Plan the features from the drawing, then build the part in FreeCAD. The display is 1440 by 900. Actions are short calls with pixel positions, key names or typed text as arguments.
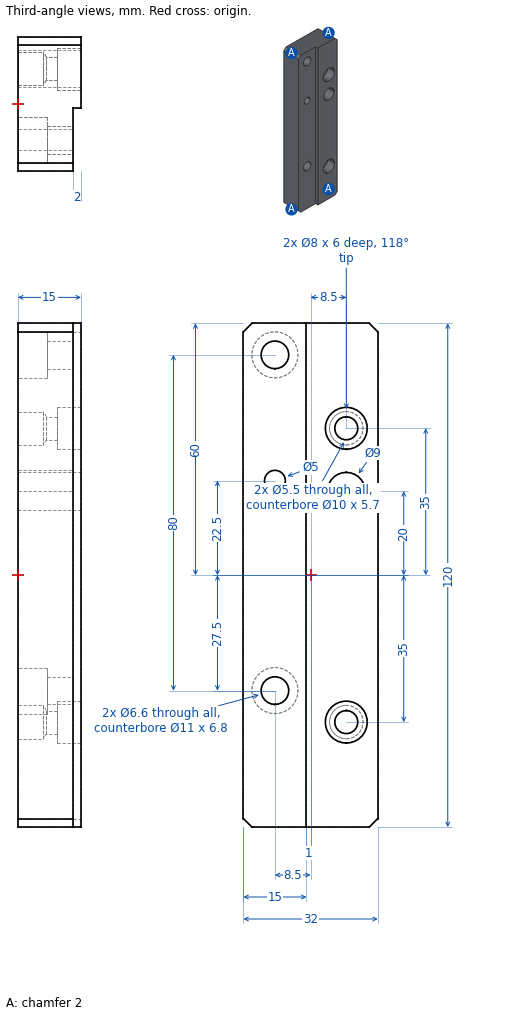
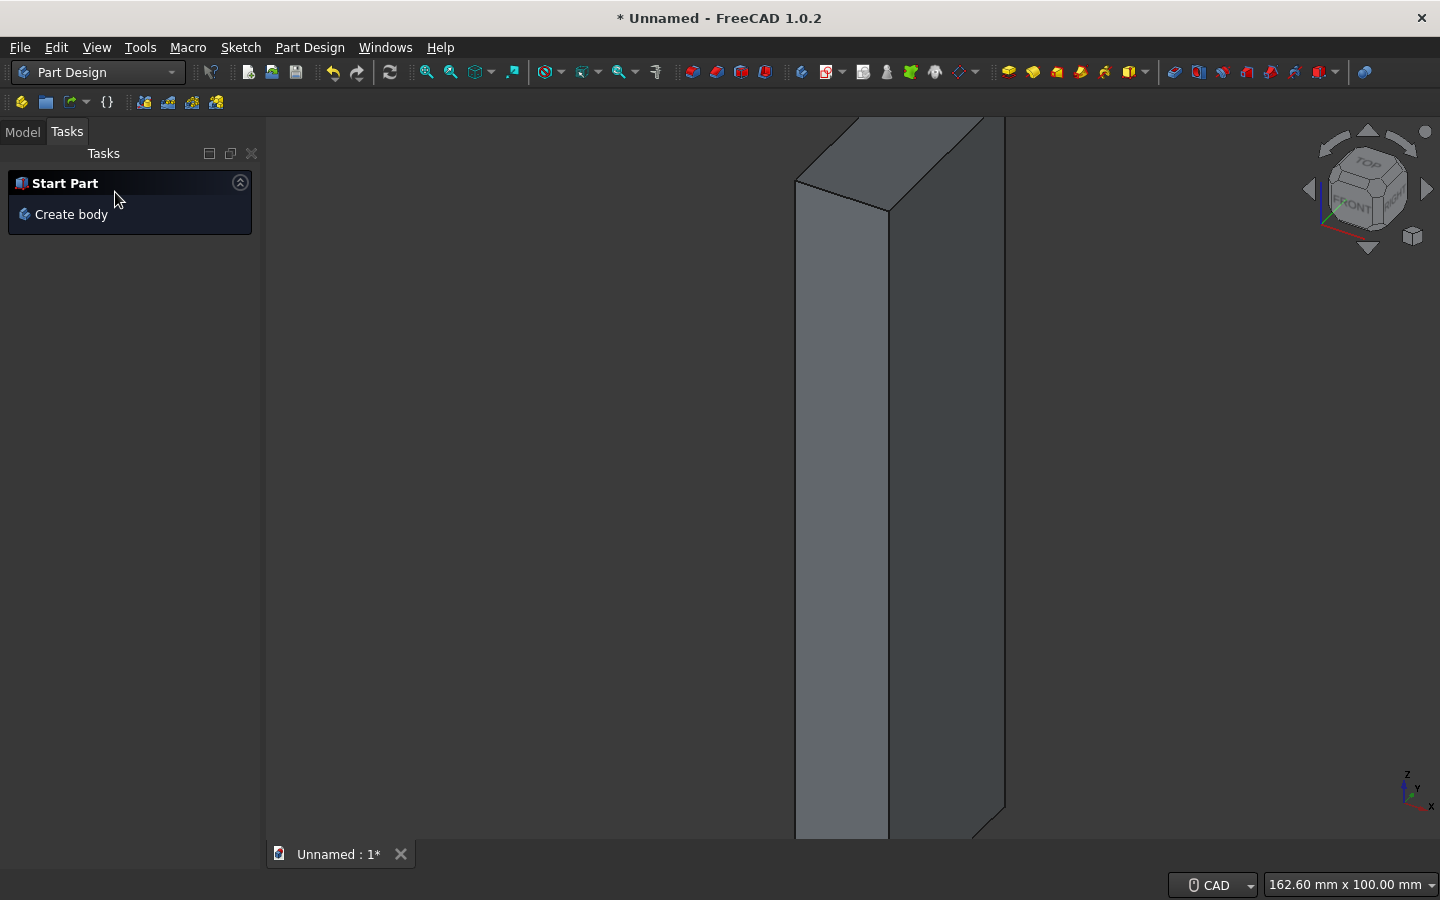
click(428, 72)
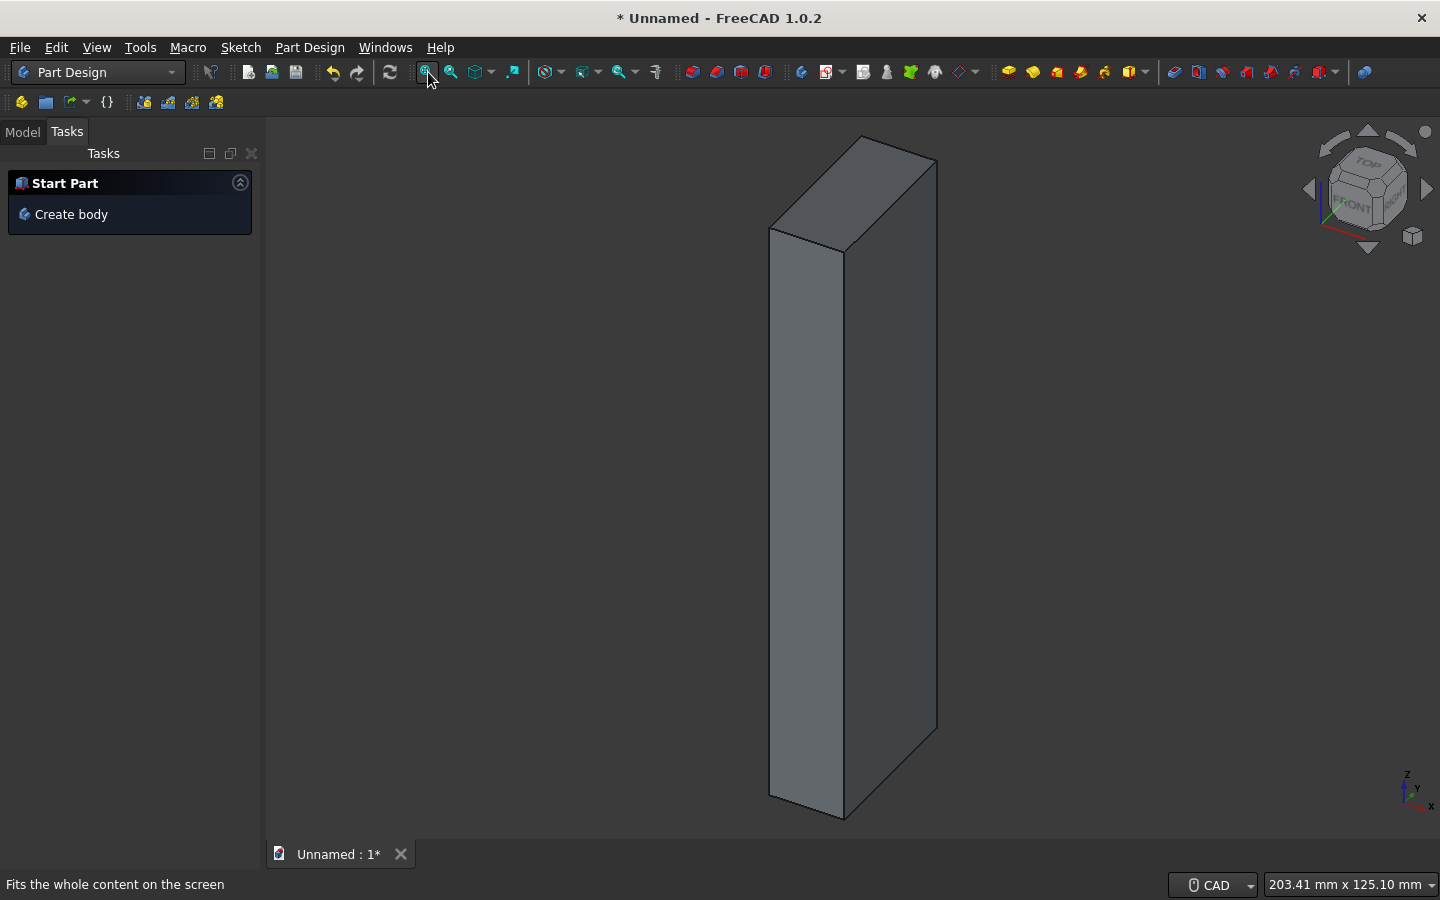
click(890, 652)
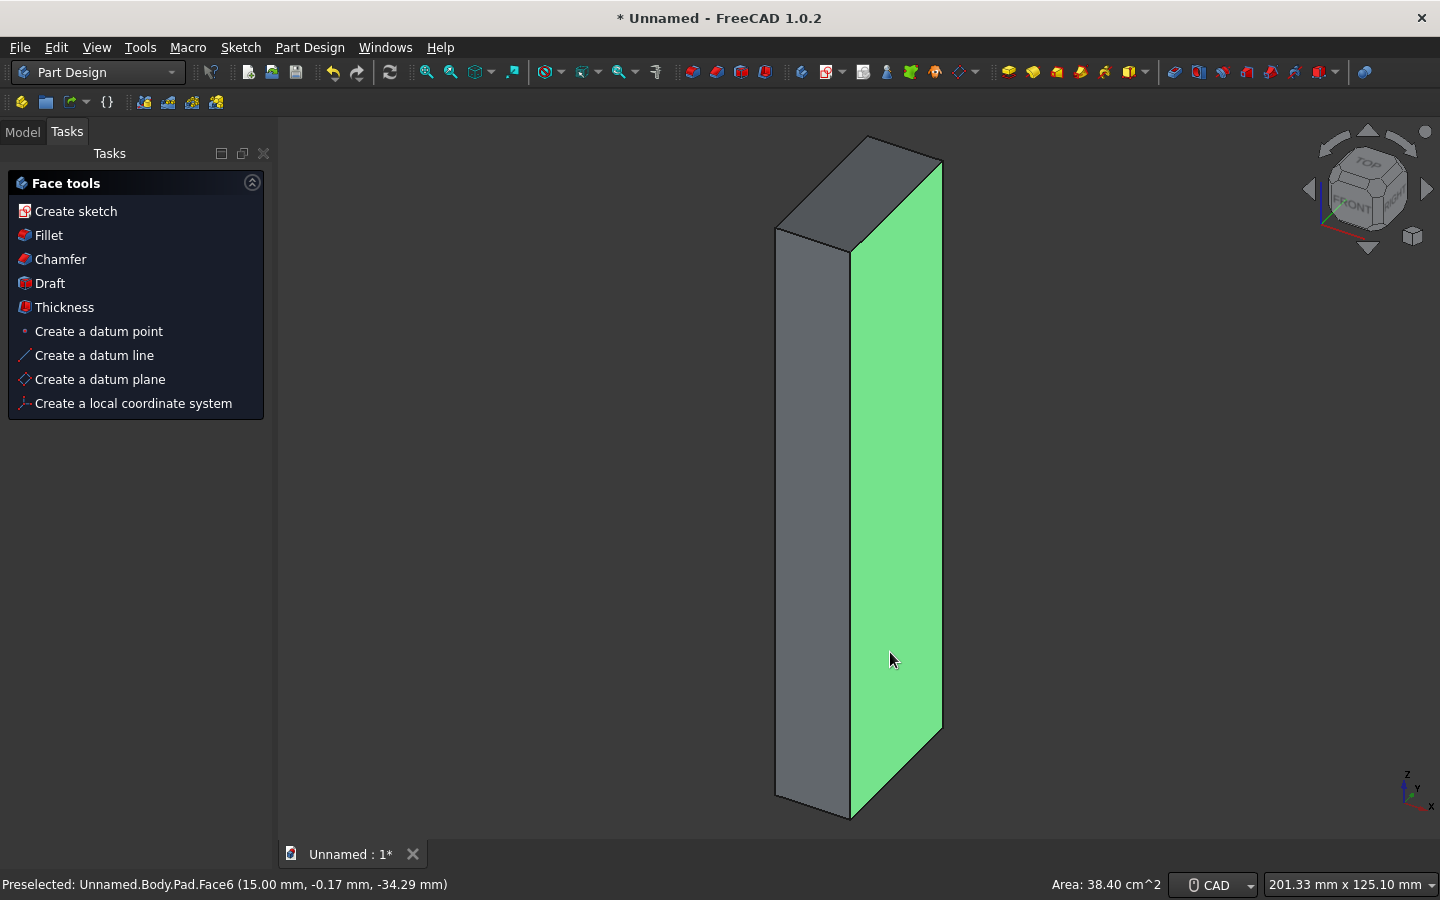
click(826, 72)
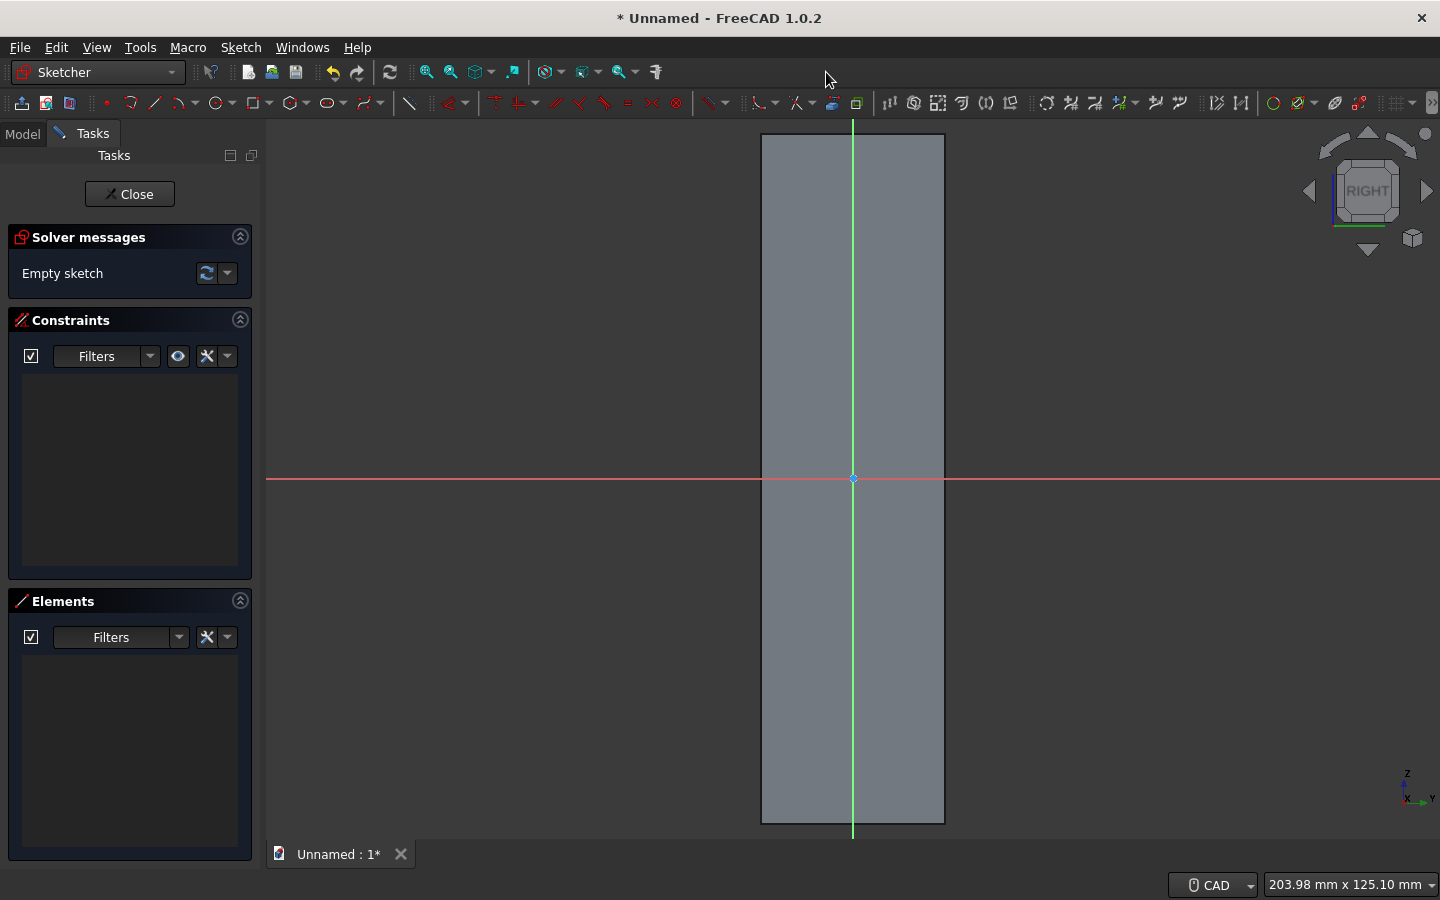
scroll(739, 479, down, 2)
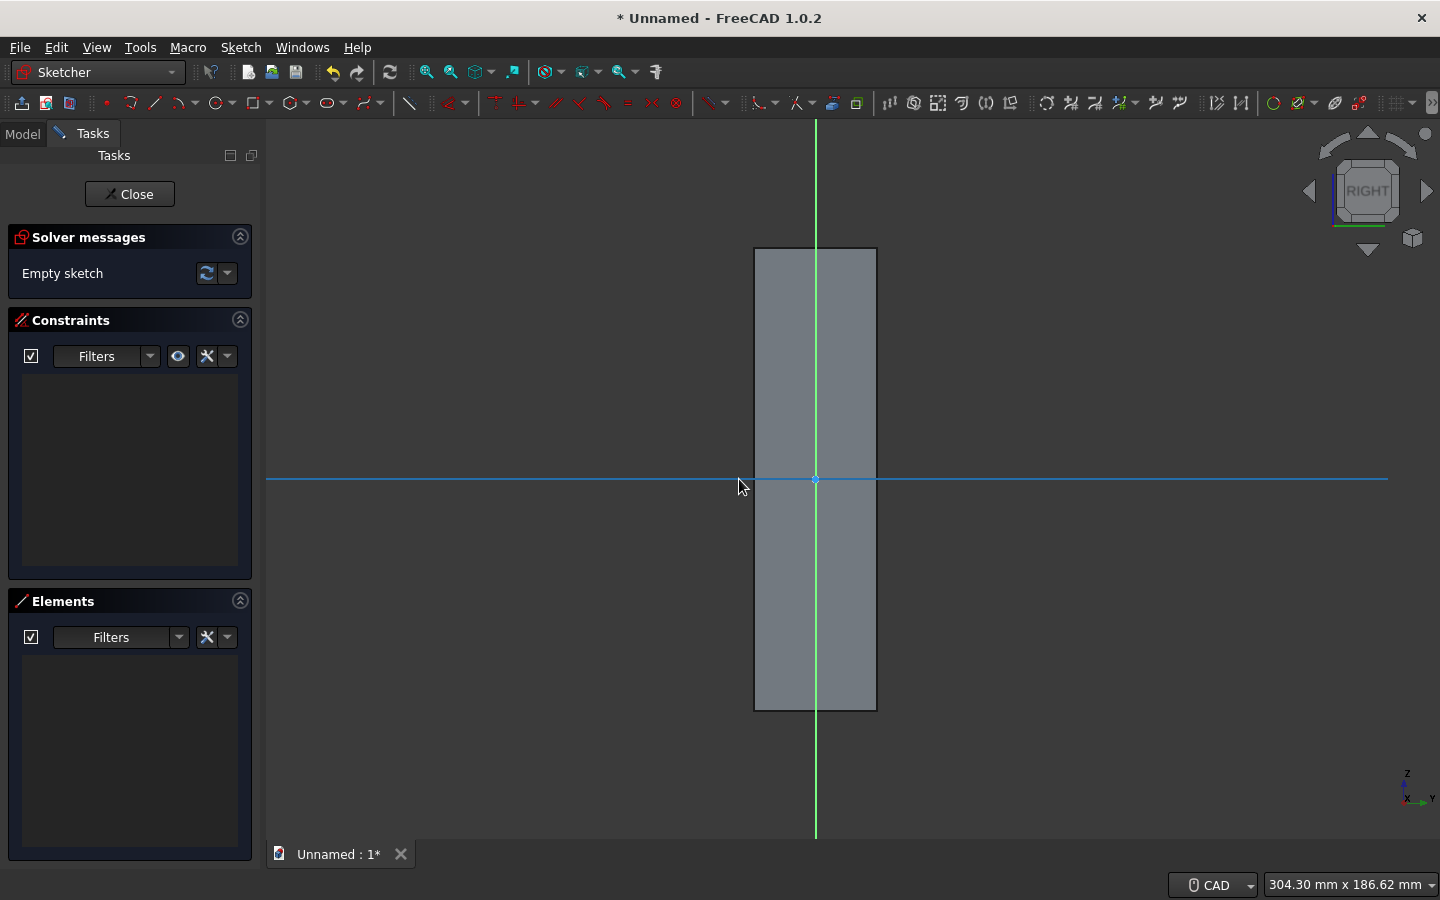
click(254, 104)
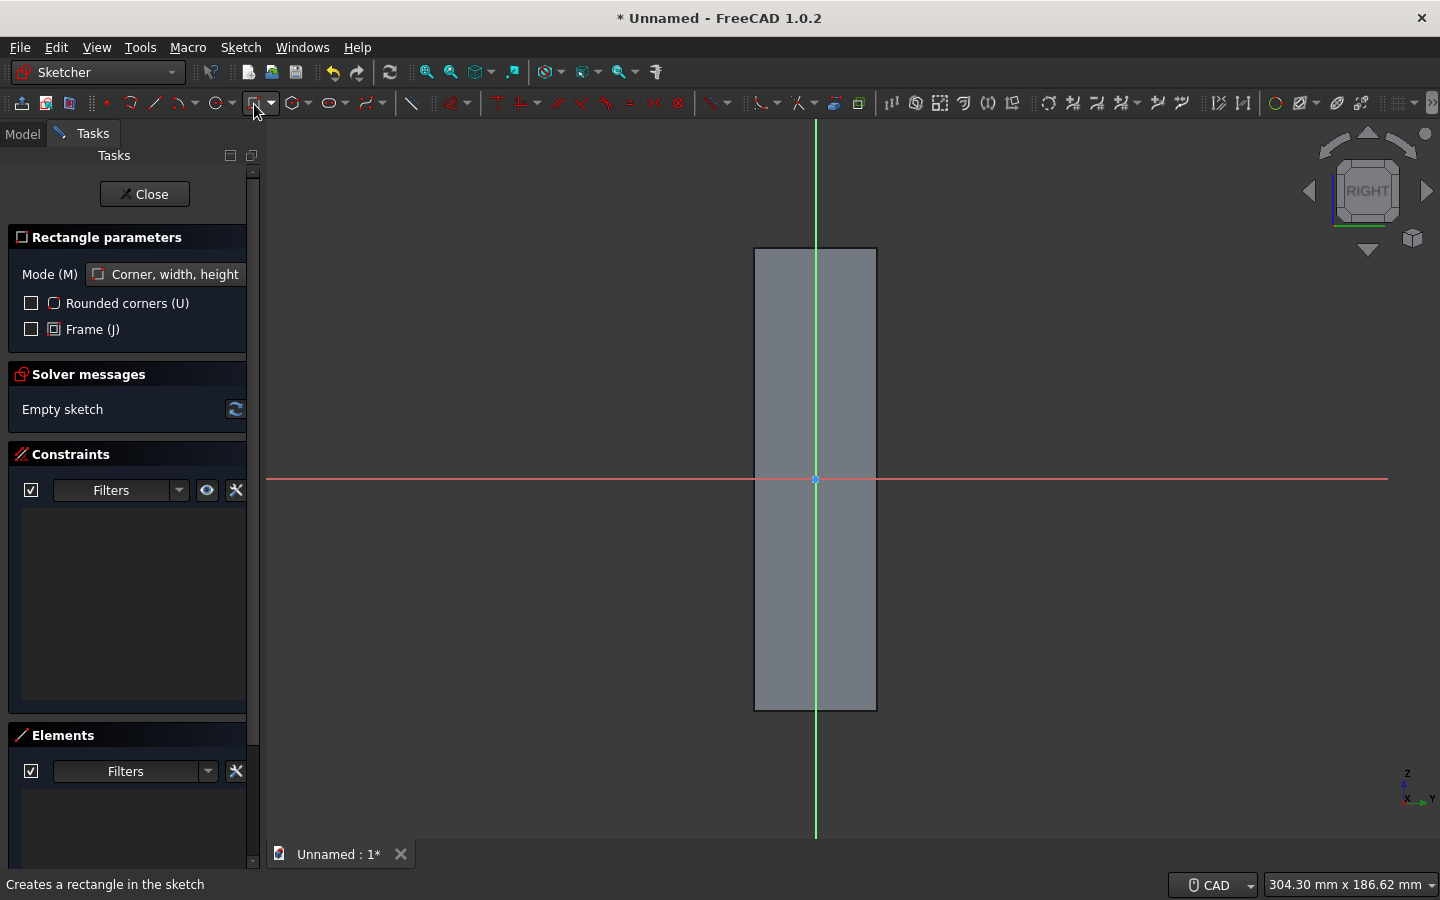
click(754, 248)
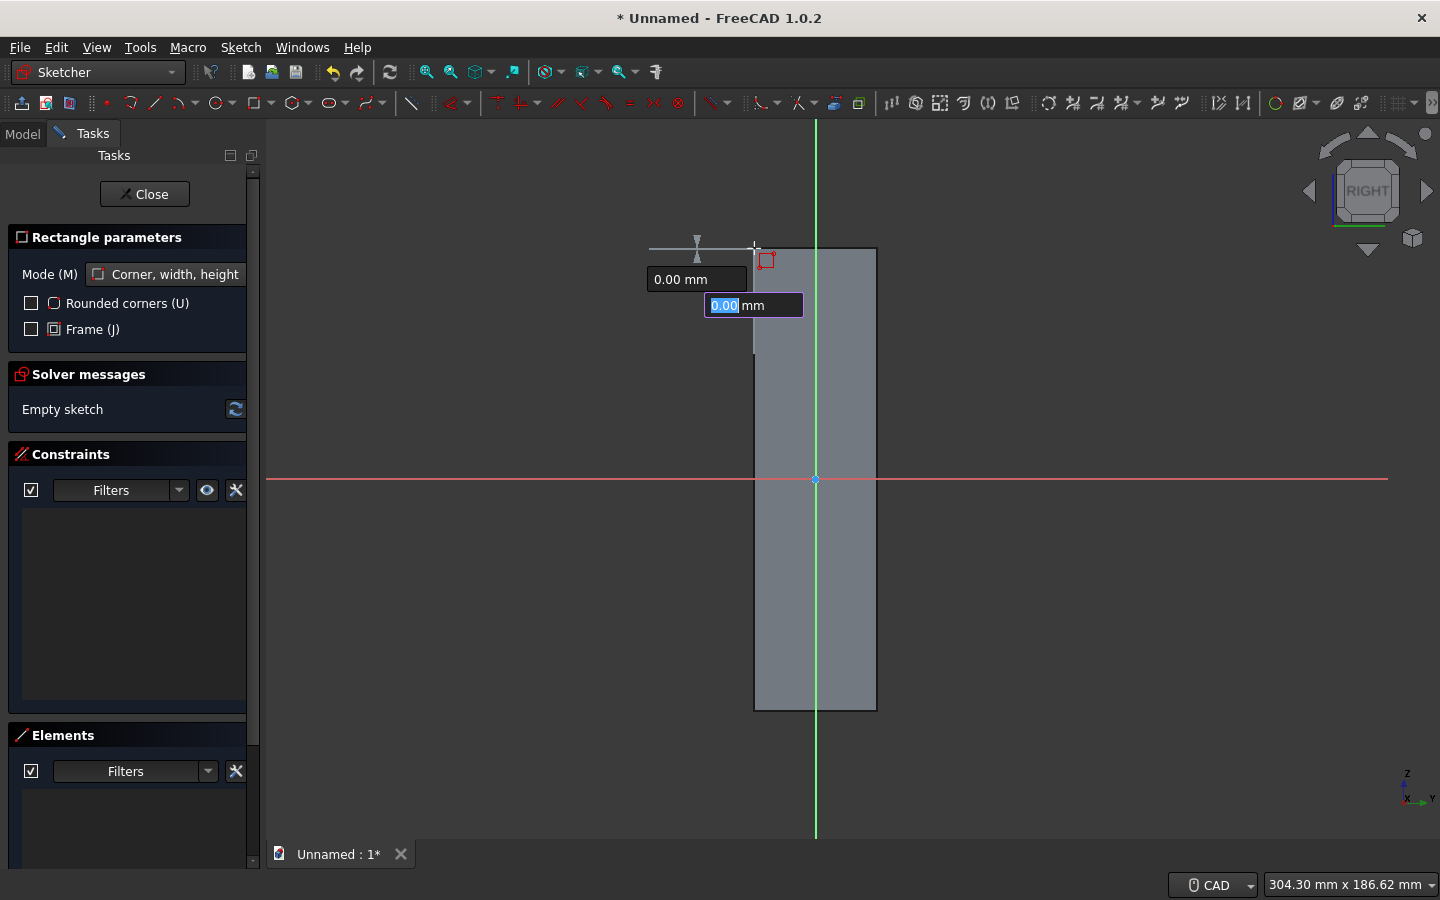
scroll(812, 711, up, 8)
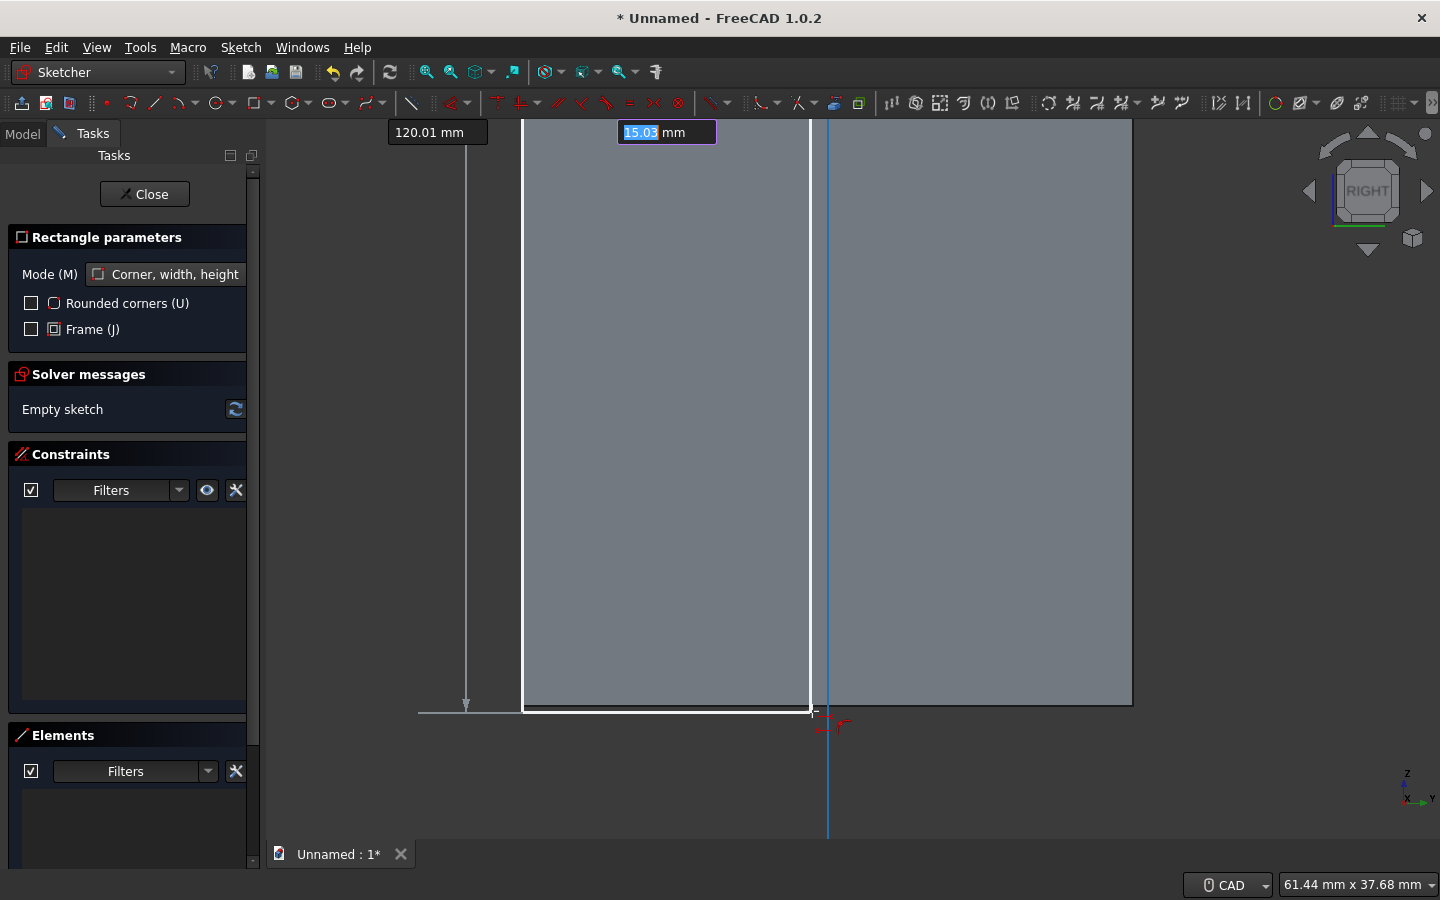
click(809, 706)
key(Escape)